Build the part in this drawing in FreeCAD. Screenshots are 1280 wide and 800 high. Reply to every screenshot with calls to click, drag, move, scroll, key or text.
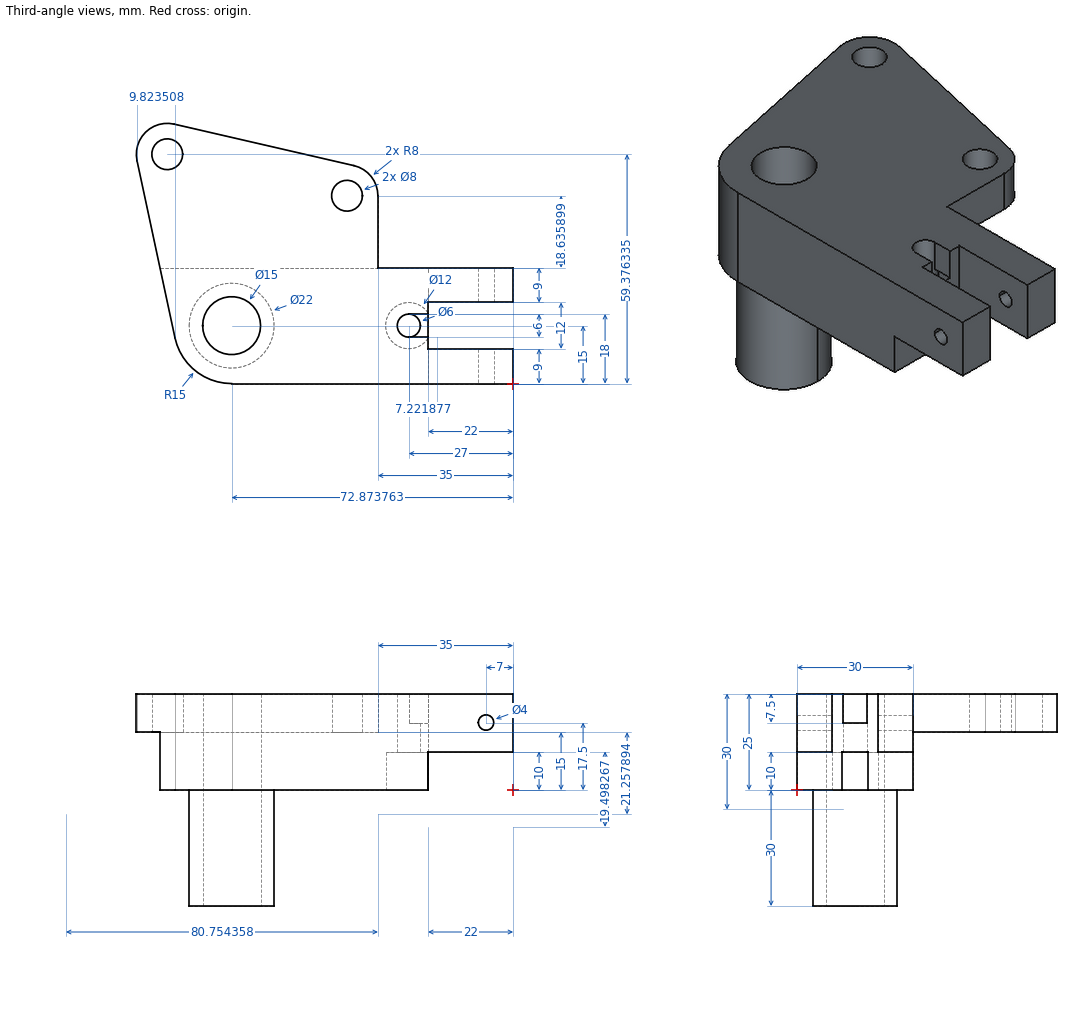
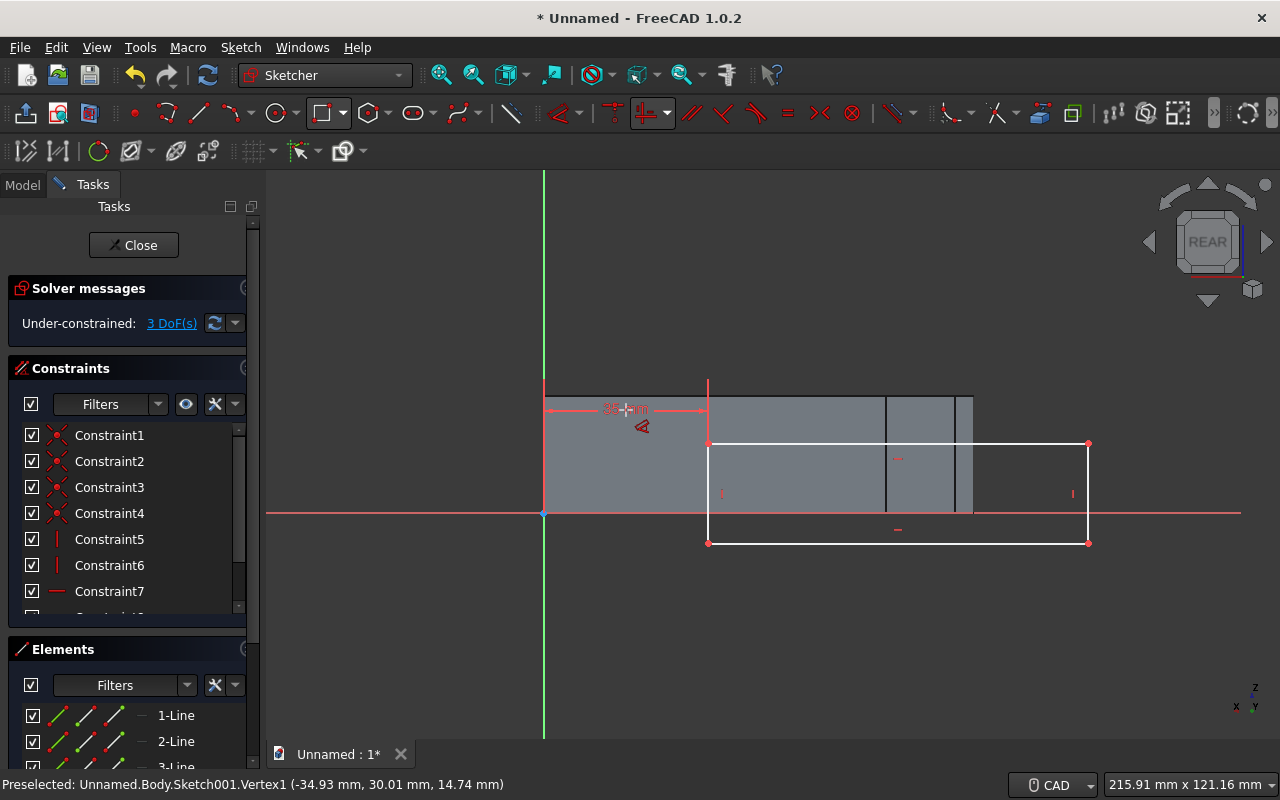
click(708, 444)
click(510, 479)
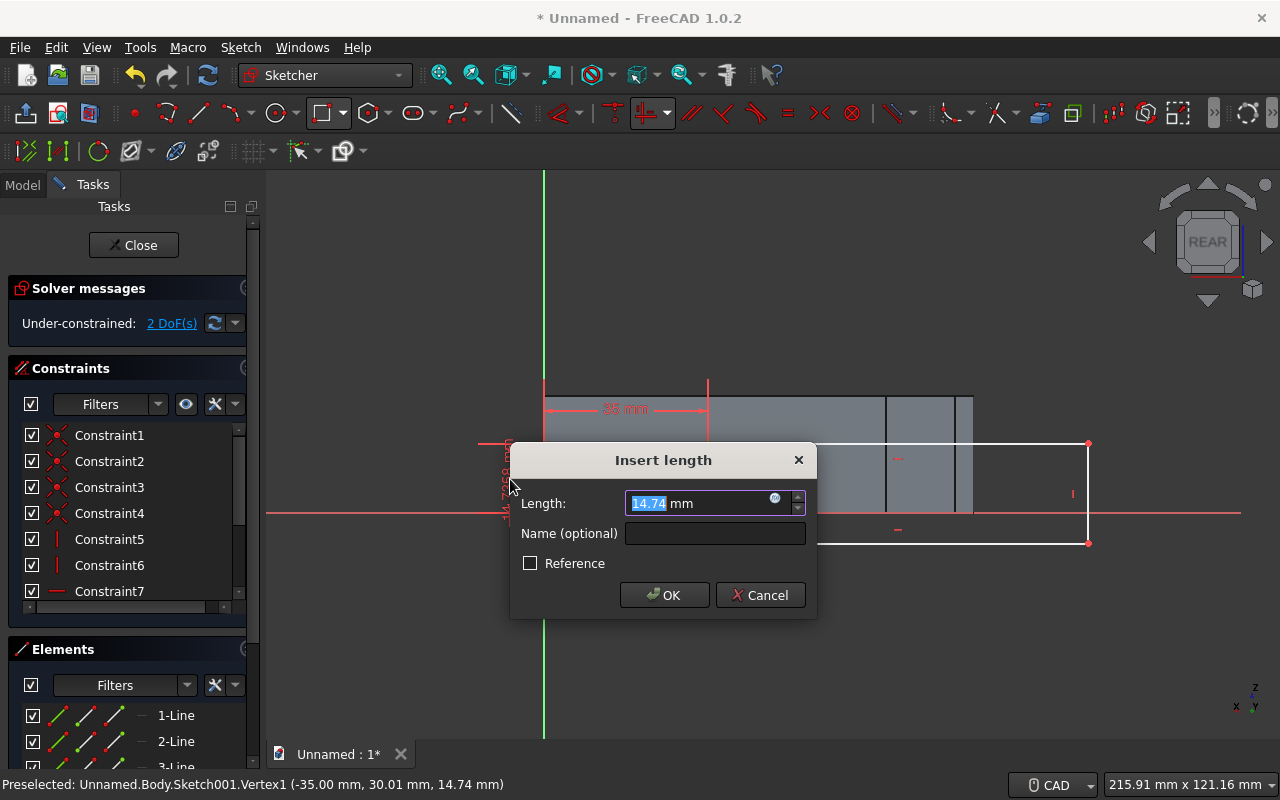
text(15)
key(Return)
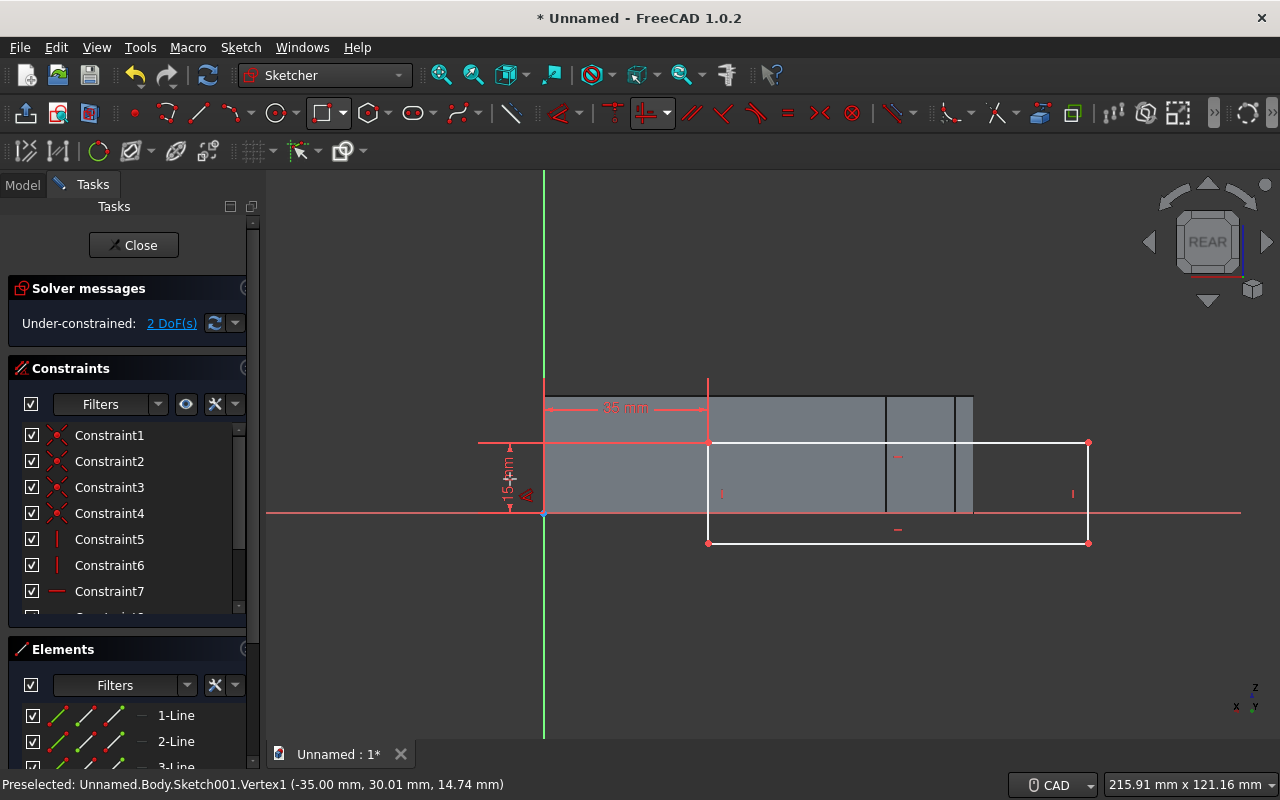
click(708, 473)
click(674, 493)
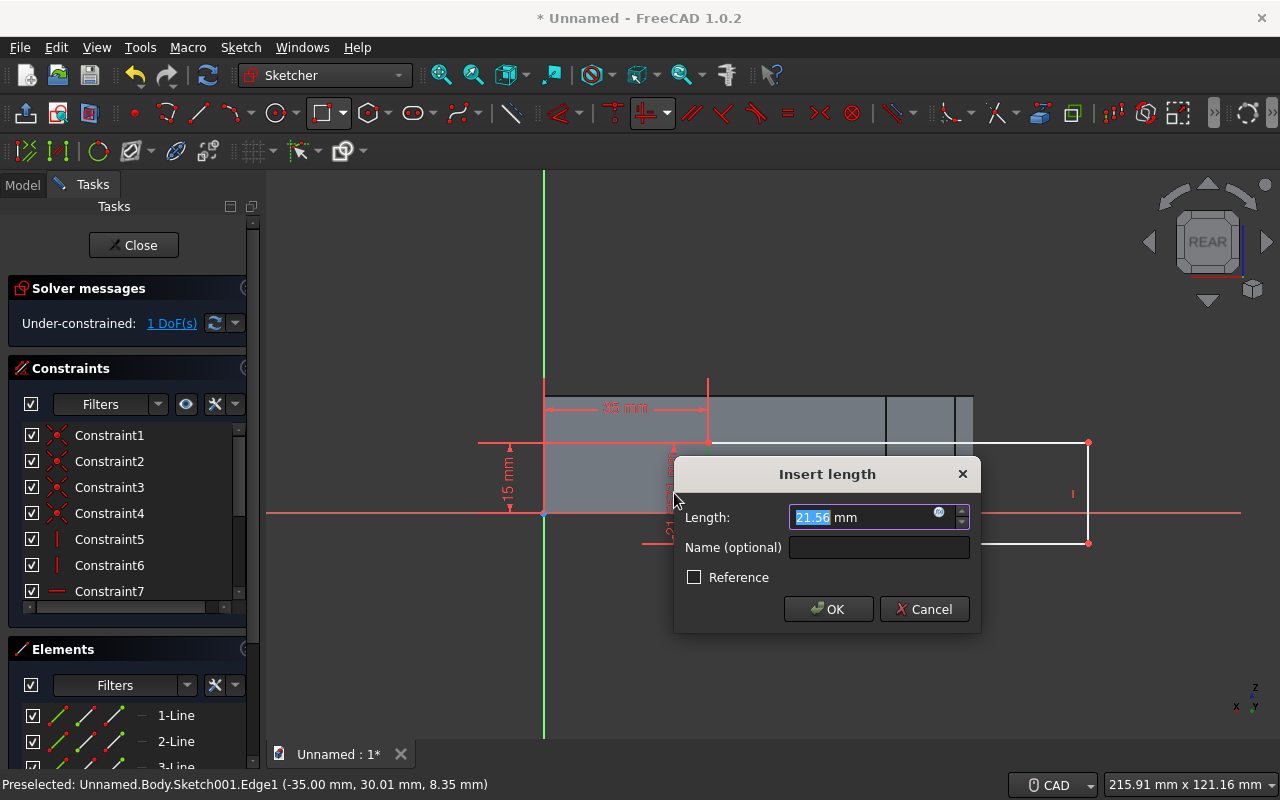
text(21.257894)
key(Return)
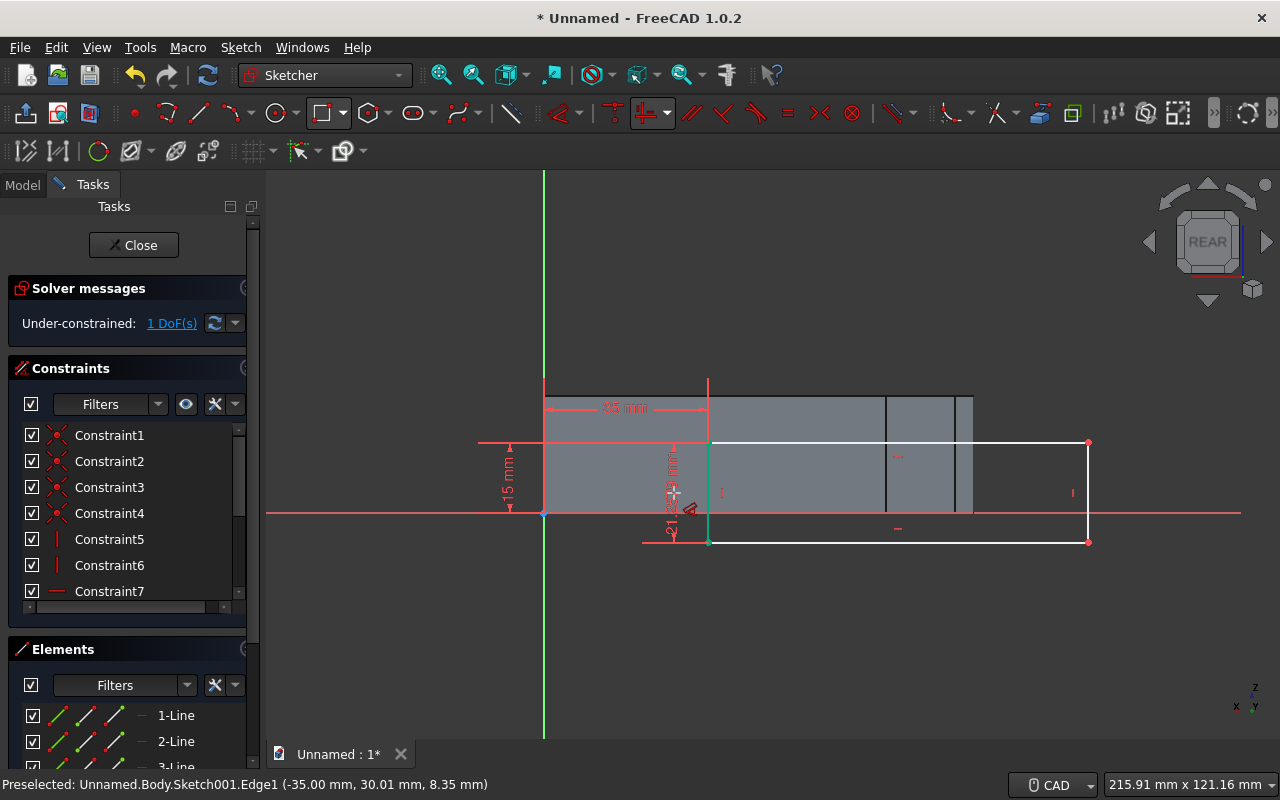
click(822, 543)
click(898, 577)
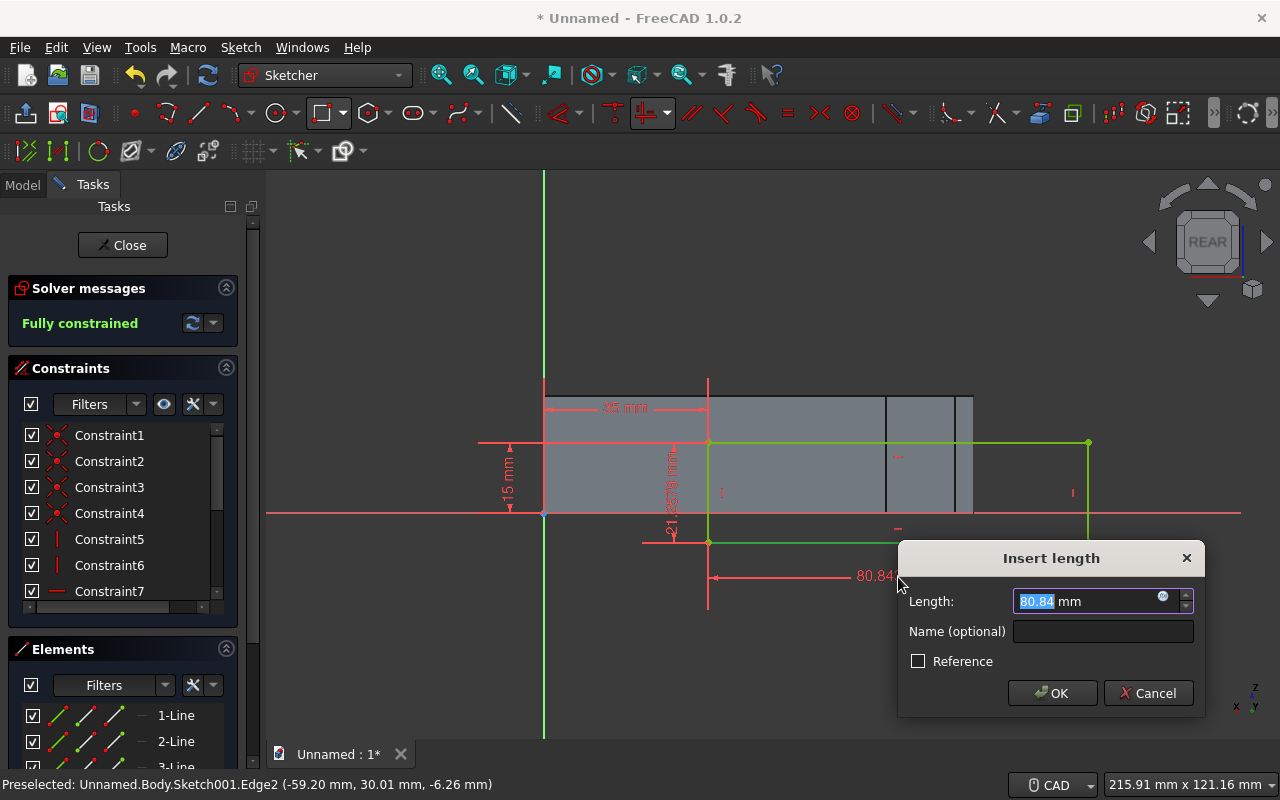
text(80.754358)
key(Return)
key(Escape)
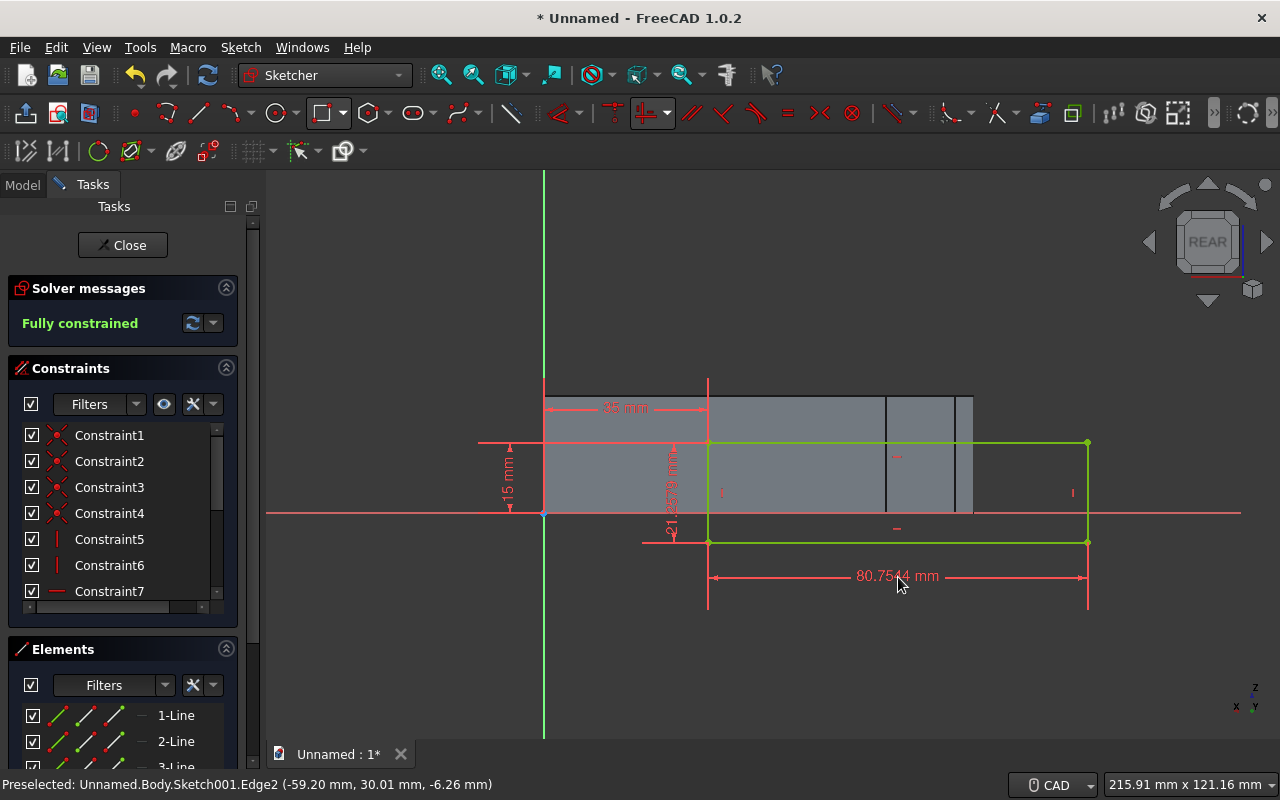
click(123, 245)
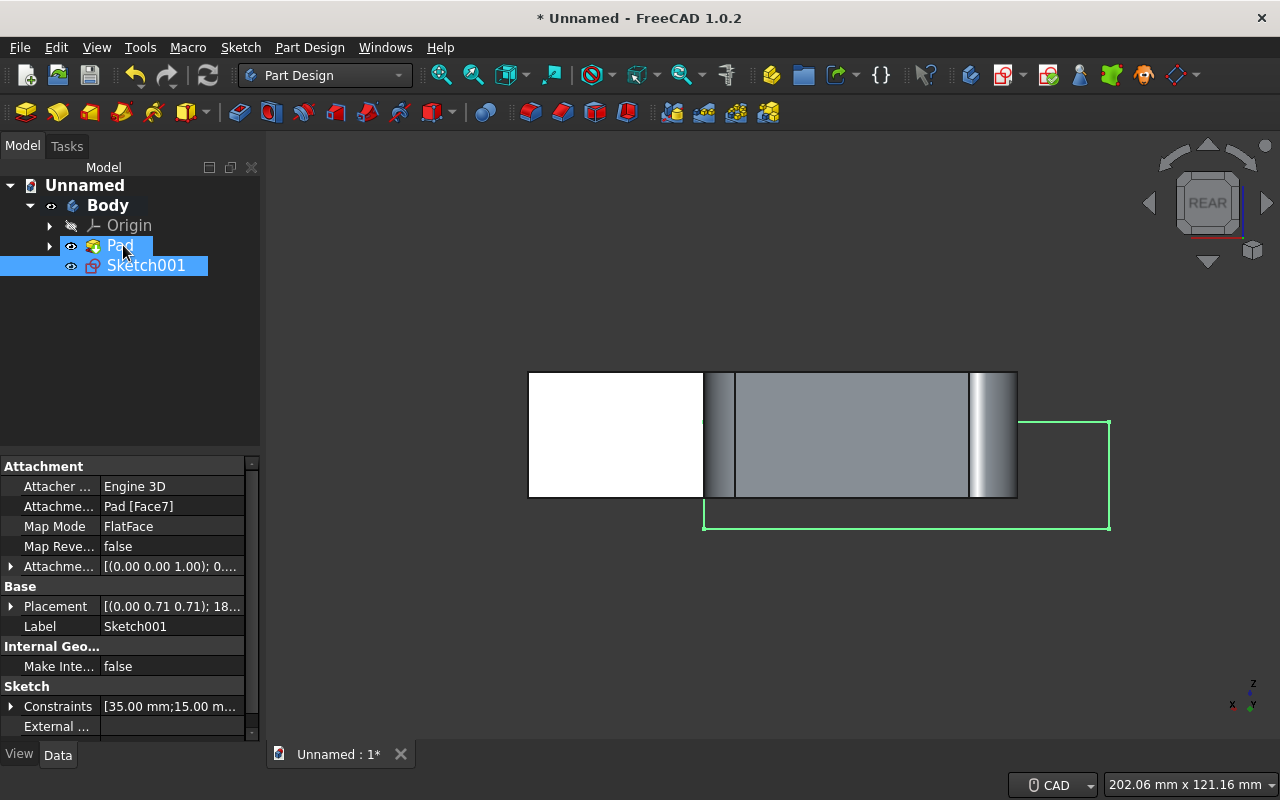
click(240, 112)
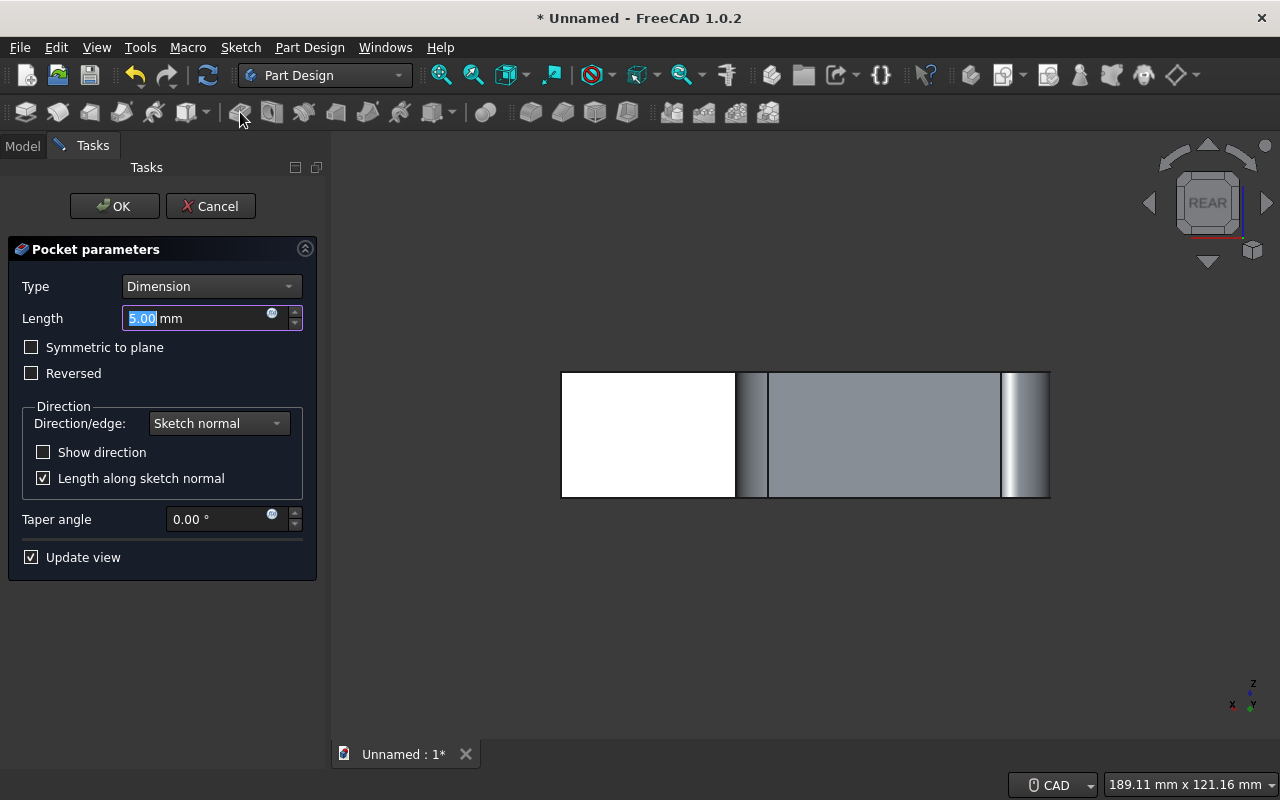
click(212, 286)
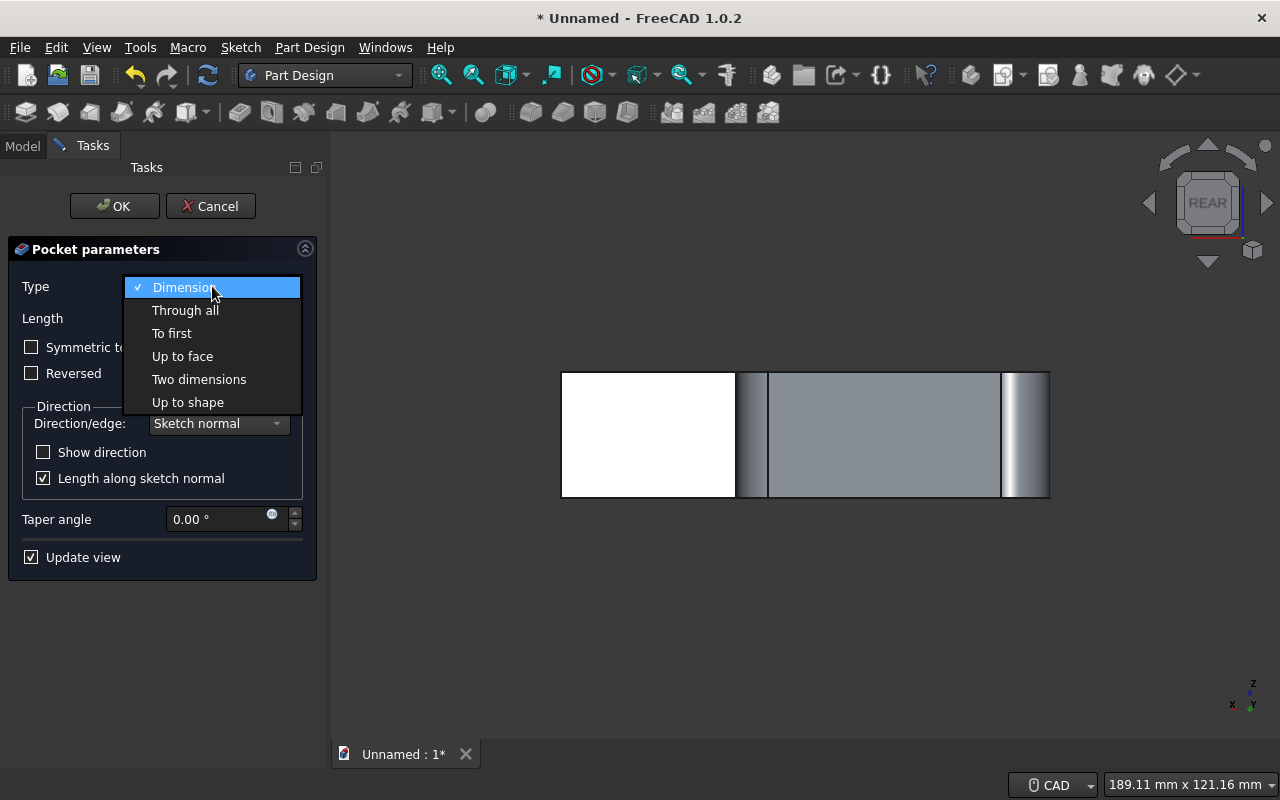
click(212, 310)